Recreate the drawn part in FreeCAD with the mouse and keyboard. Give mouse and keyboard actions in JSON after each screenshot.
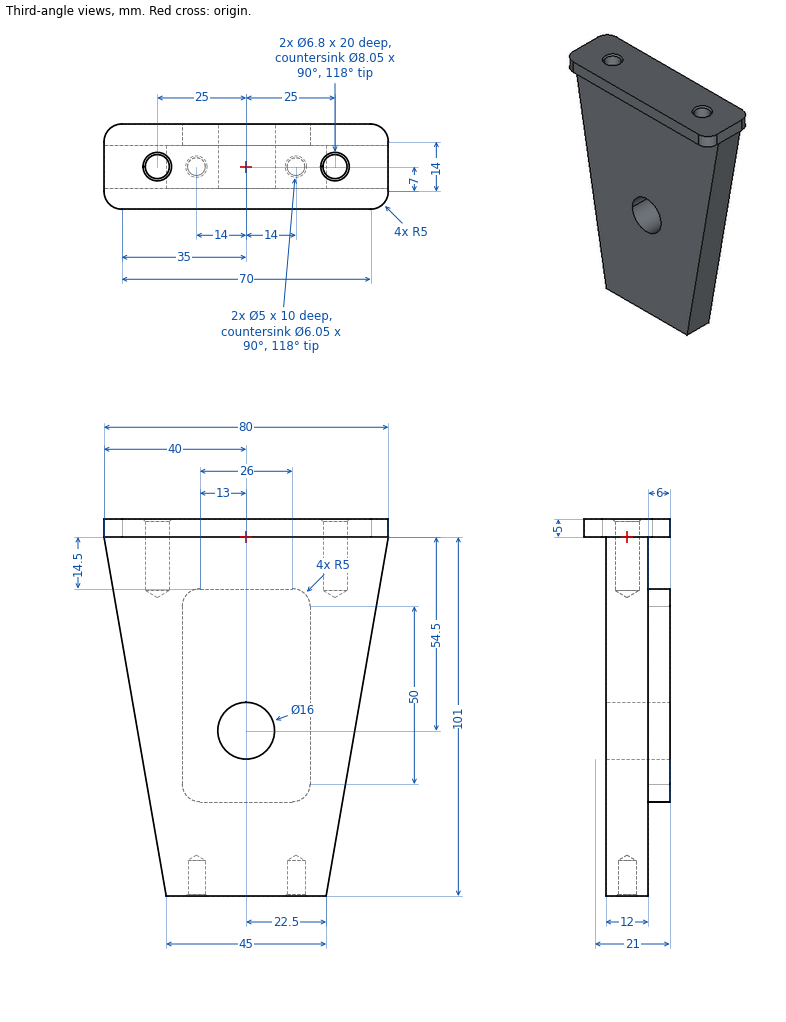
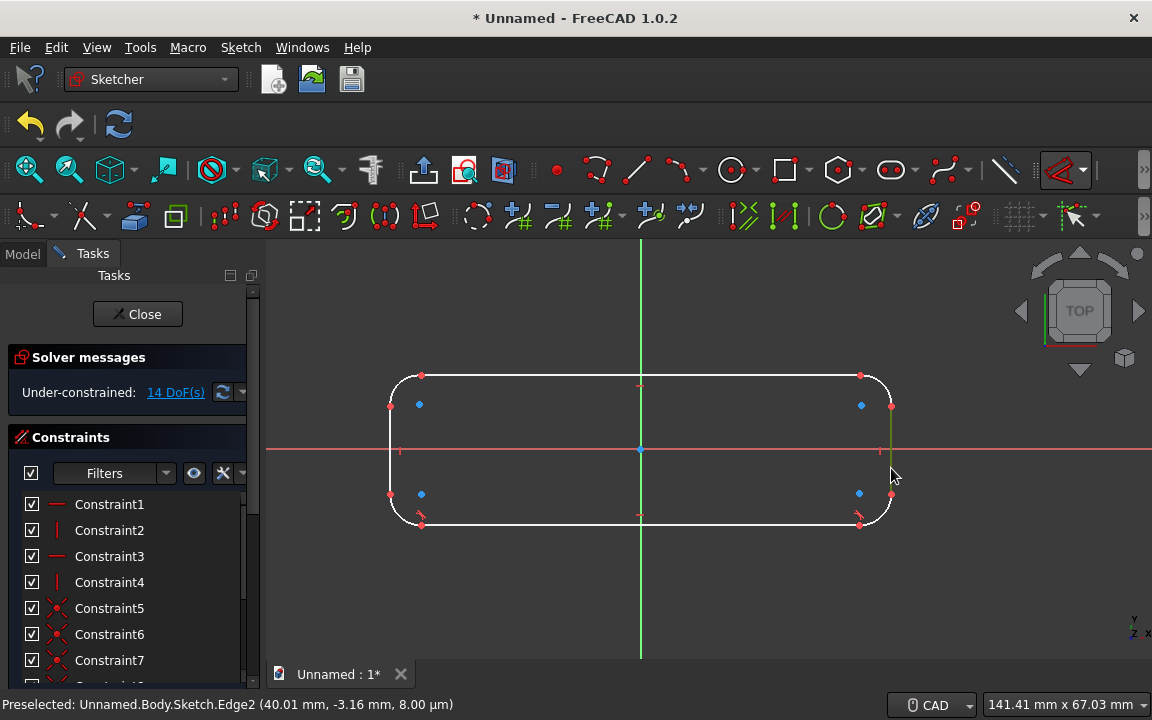
{"action": "left_click", "coordinate": [873, 522]}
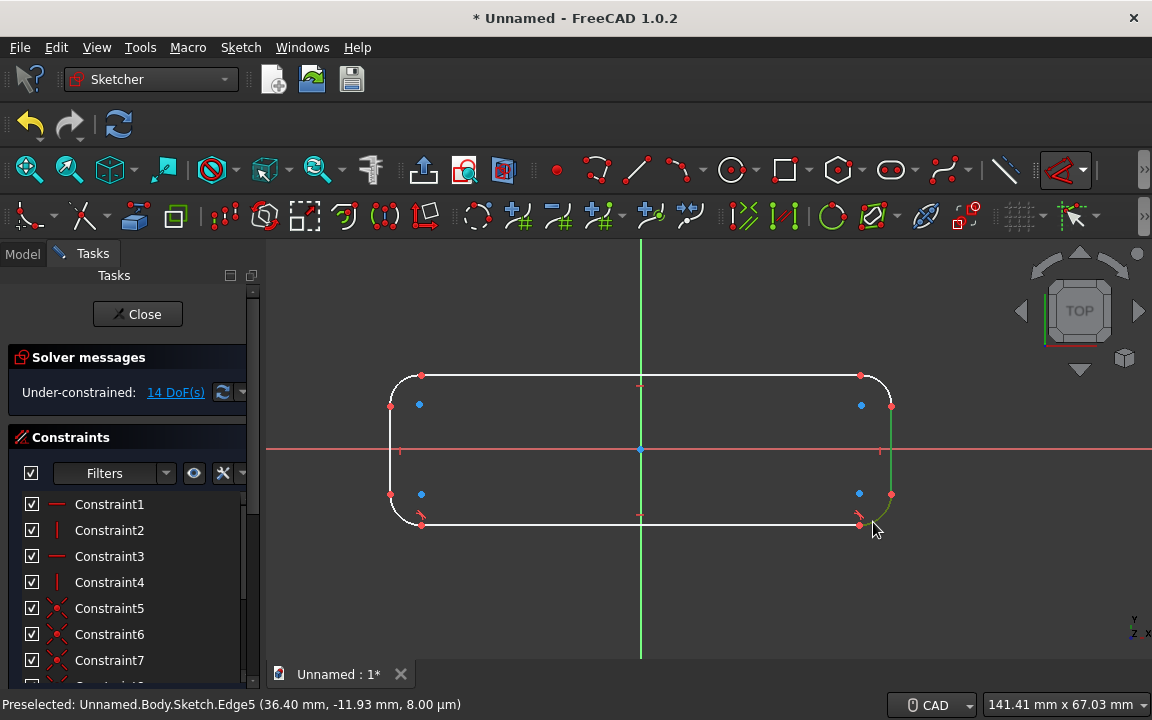
{"action": "key", "text": "t"}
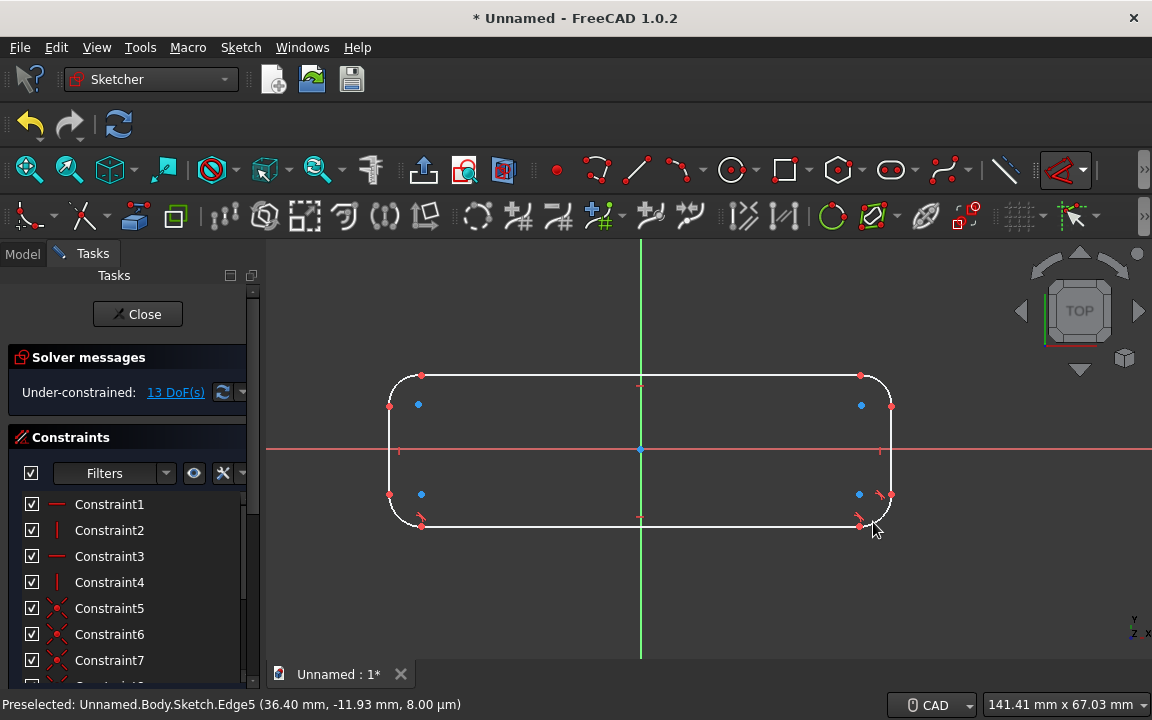
{"action": "left_click", "coordinate": [891, 468]}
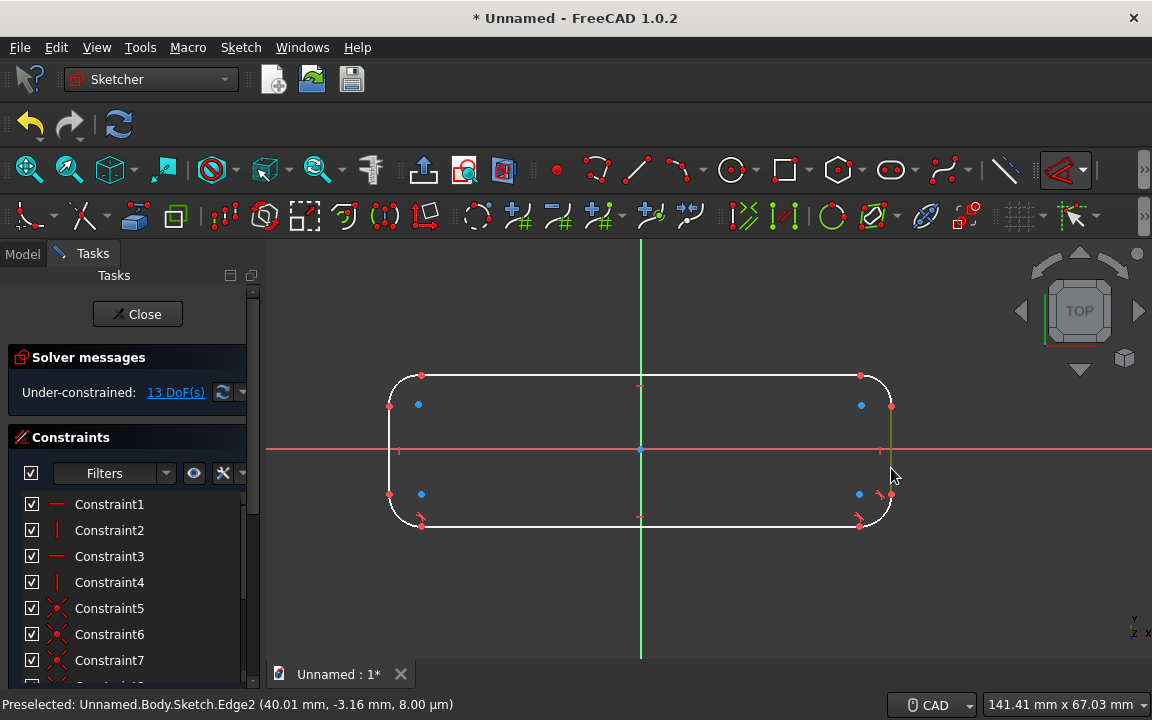
{"action": "left_click", "coordinate": [888, 392]}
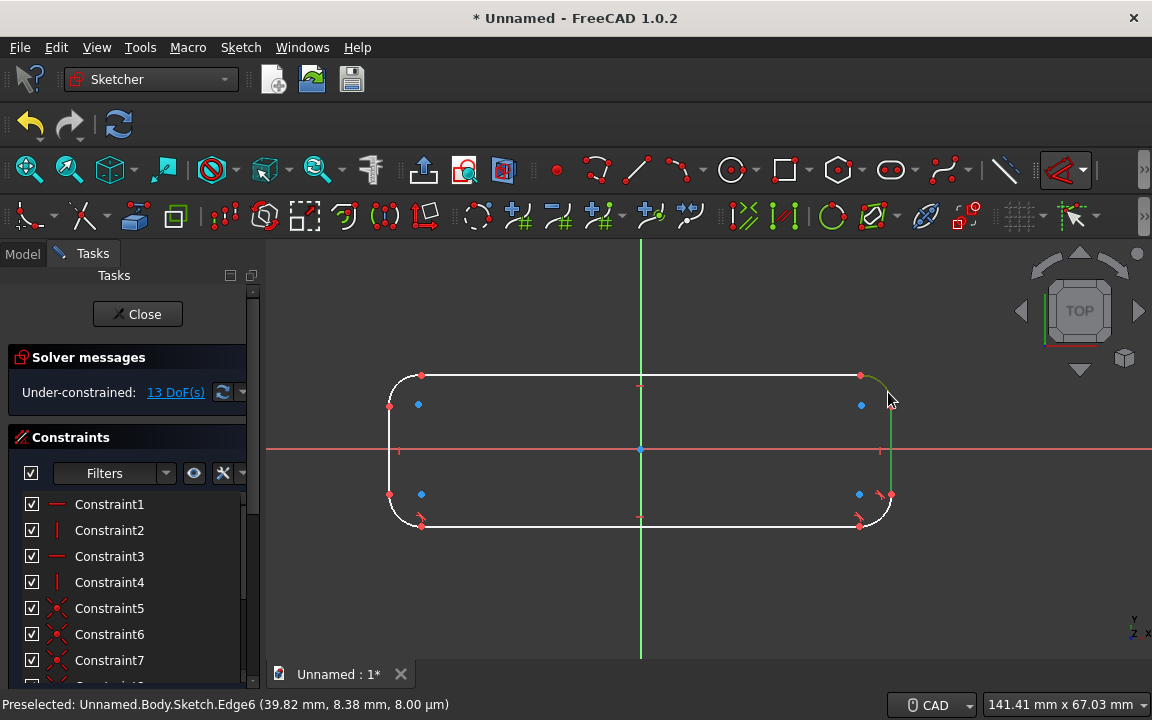
{"action": "key", "text": "t"}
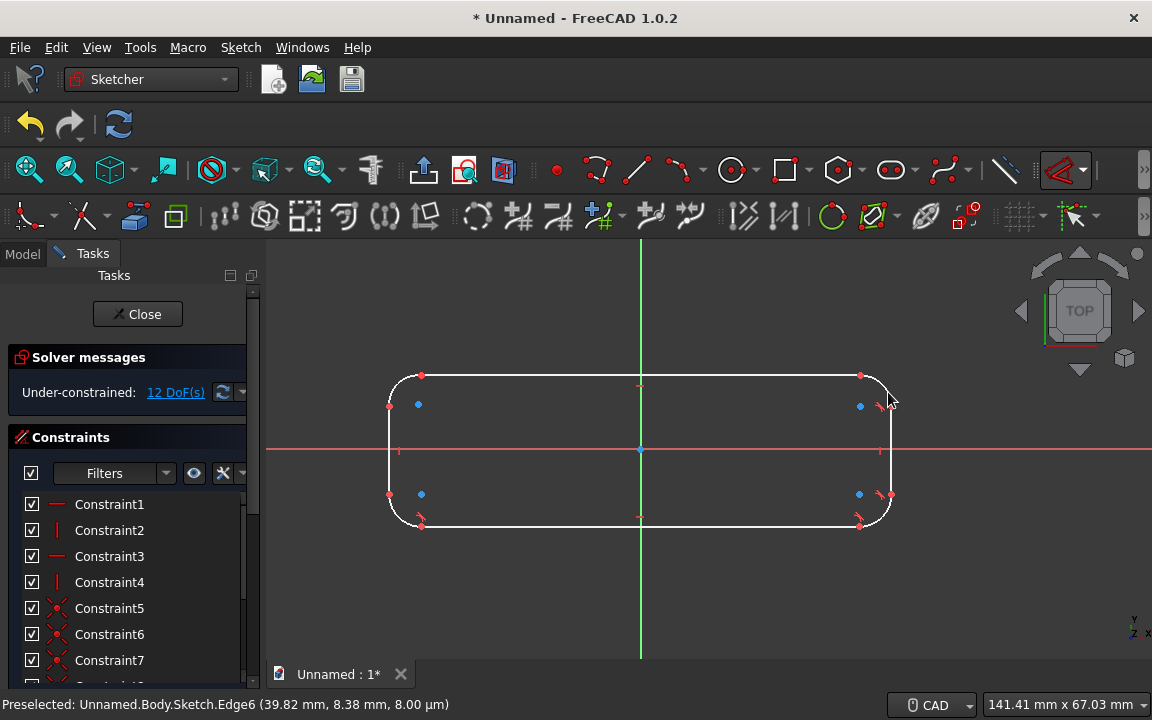
{"action": "left_click", "coordinate": [729, 375]}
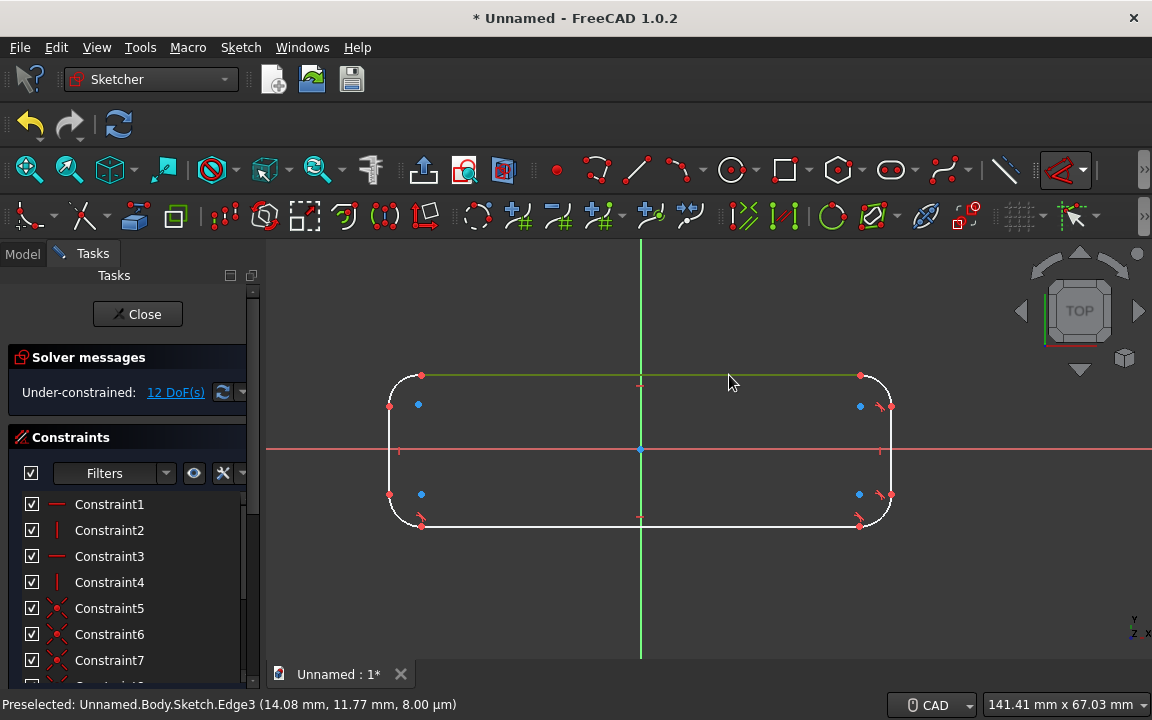
{"action": "left_click", "coordinate": [888, 392]}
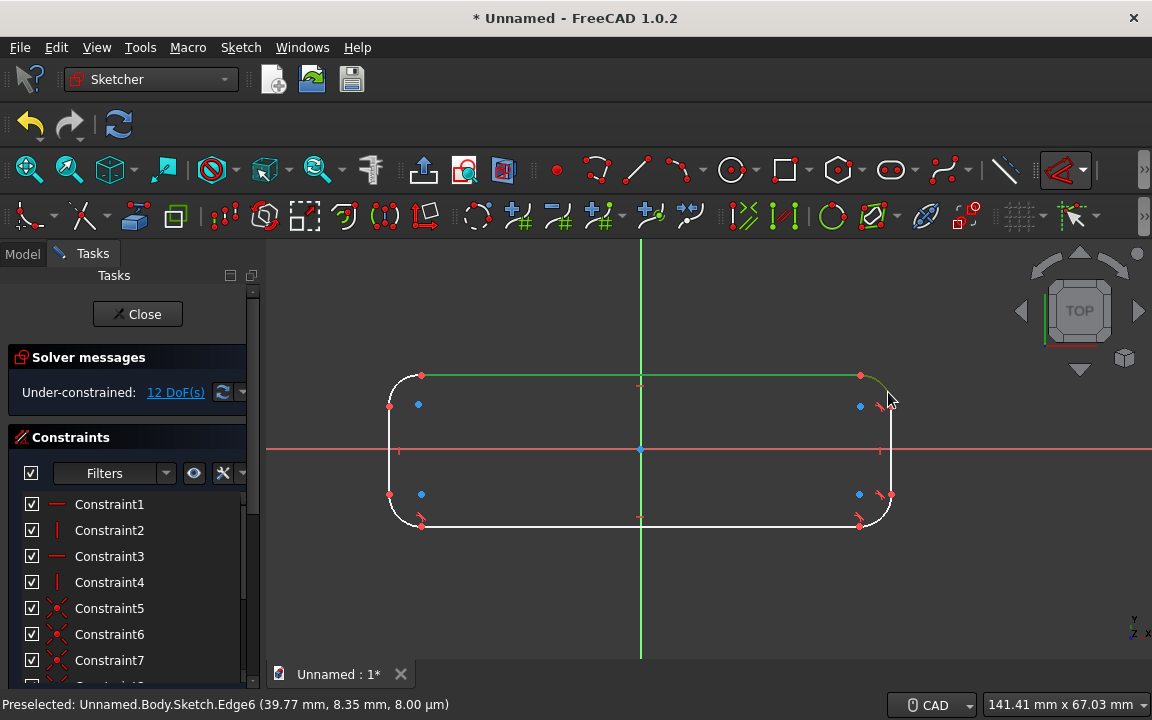
{"action": "key", "text": "t"}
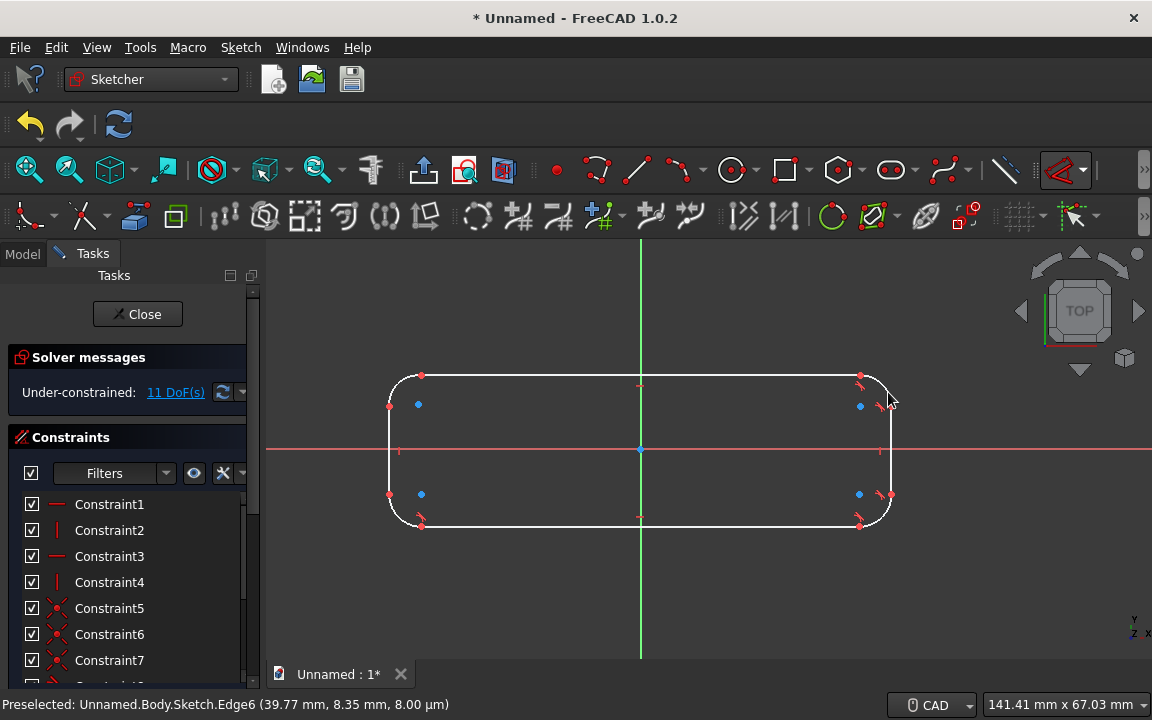
{"action": "left_click", "coordinate": [729, 375]}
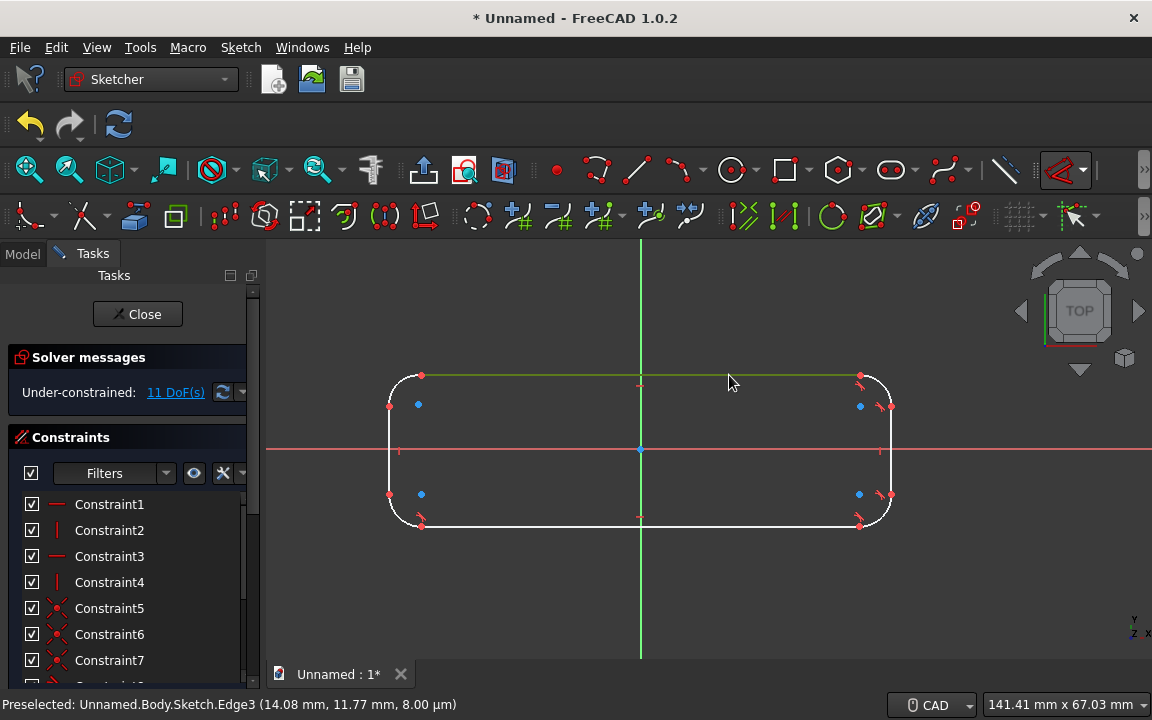
{"action": "left_click", "coordinate": [407, 378]}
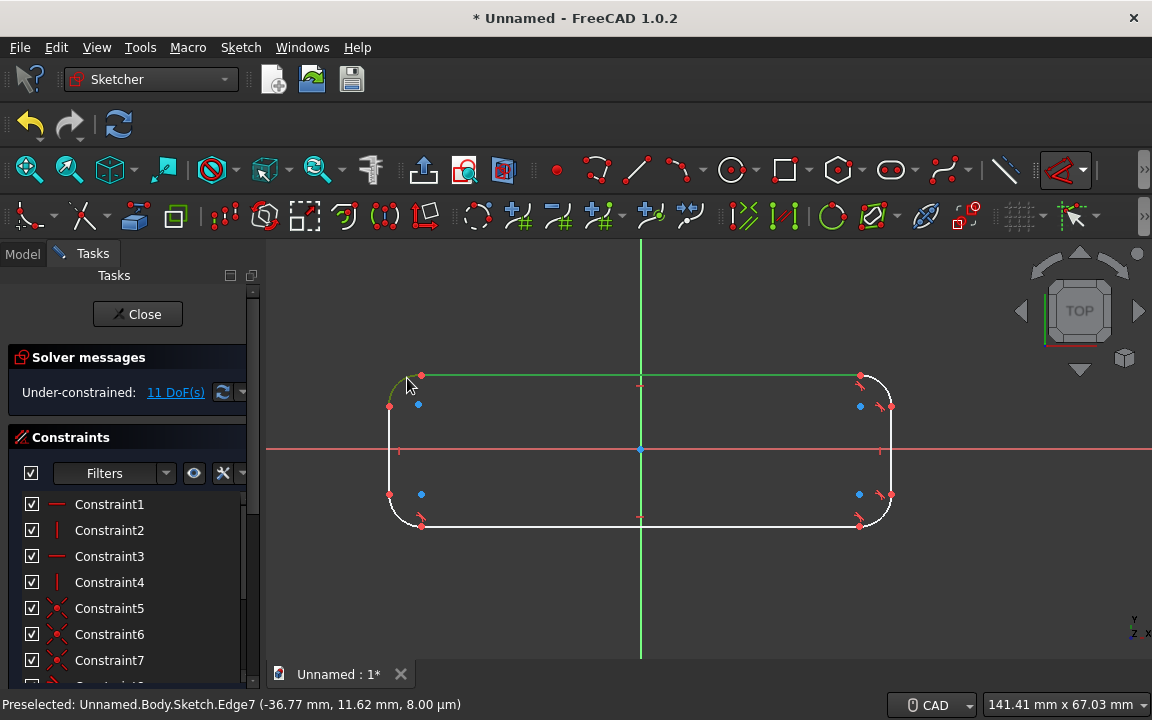
{"action": "key", "text": "t"}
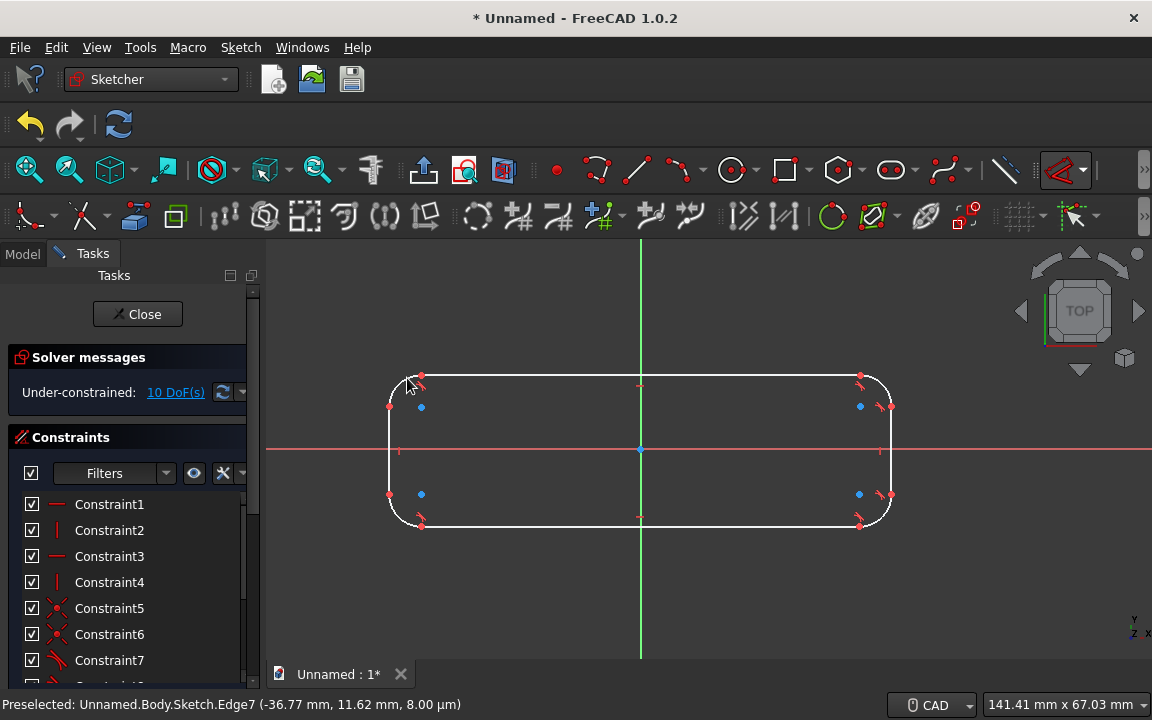
{"action": "left_click", "coordinate": [389, 433]}